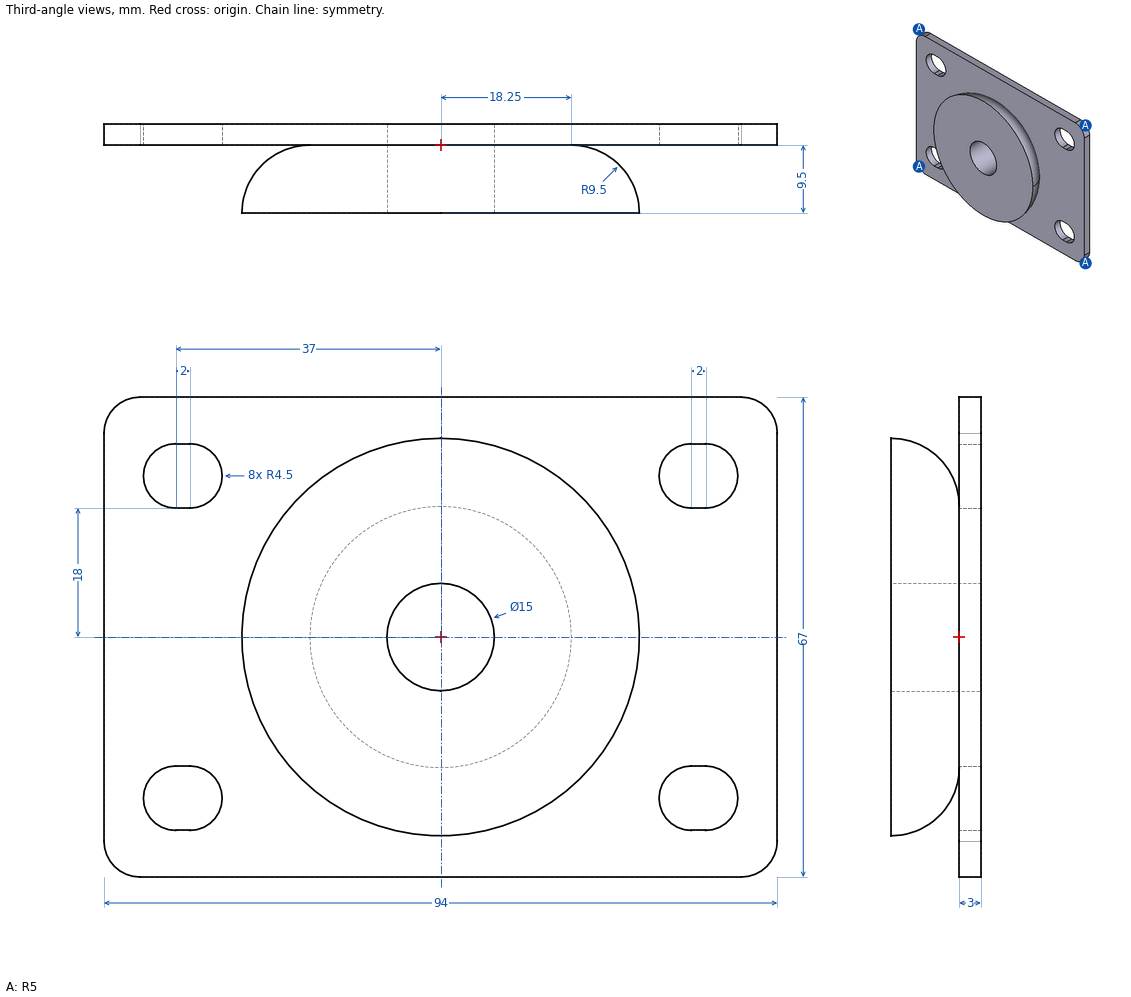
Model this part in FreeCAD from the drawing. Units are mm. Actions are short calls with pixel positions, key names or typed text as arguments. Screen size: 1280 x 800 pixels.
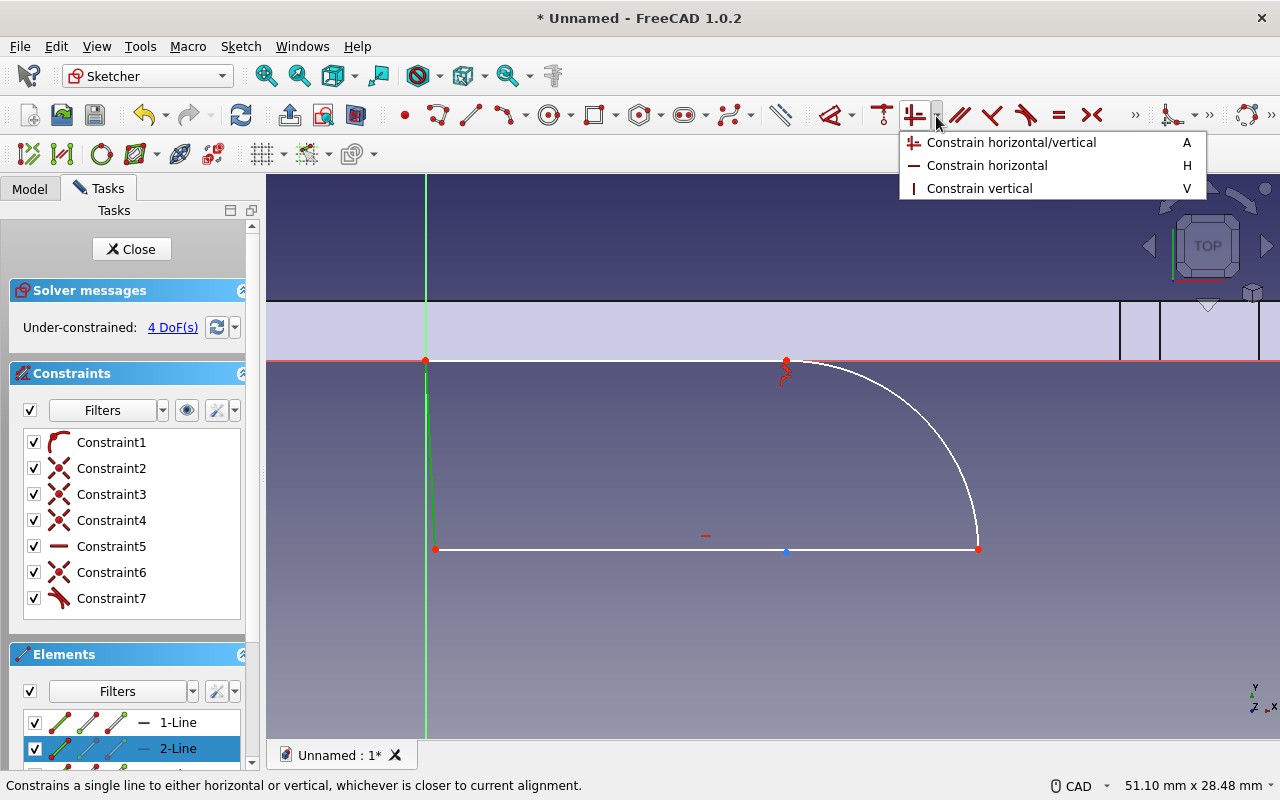
click(1053, 188)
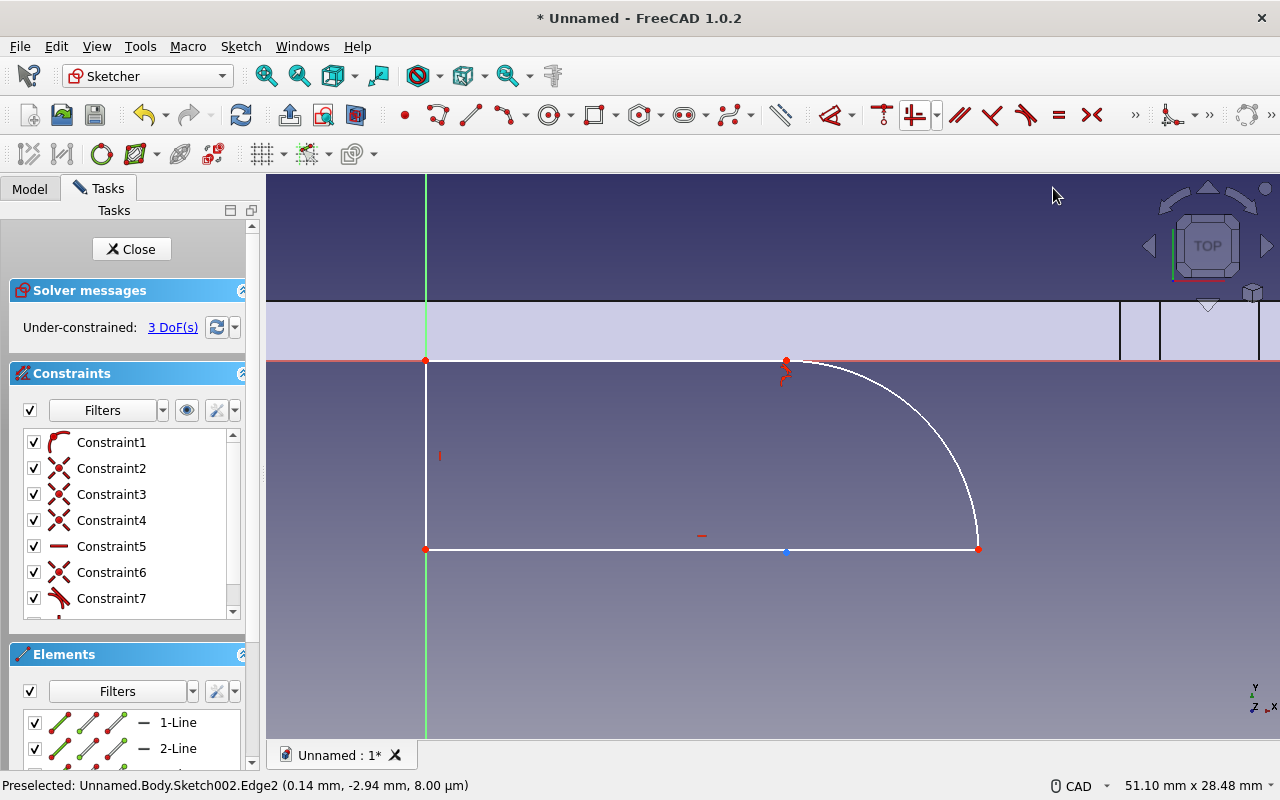
key(d)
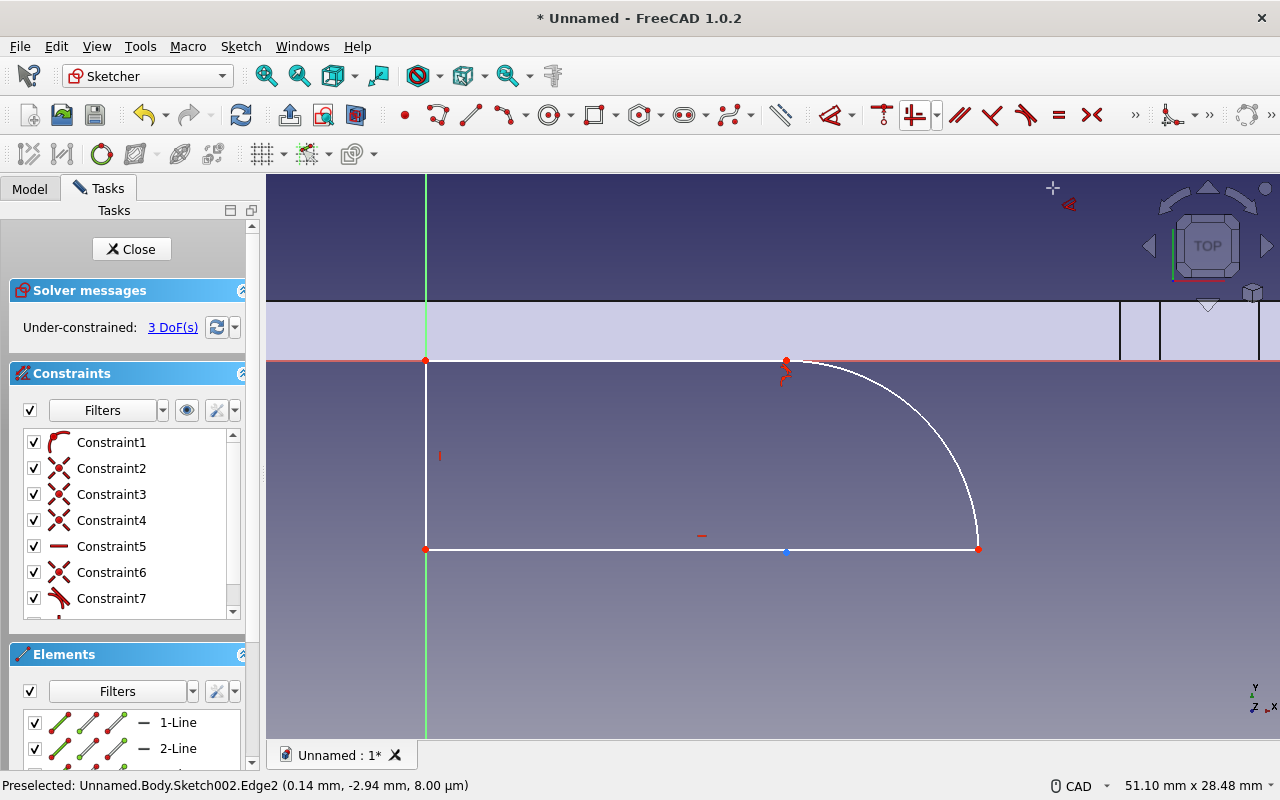
click(957, 464)
click(985, 449)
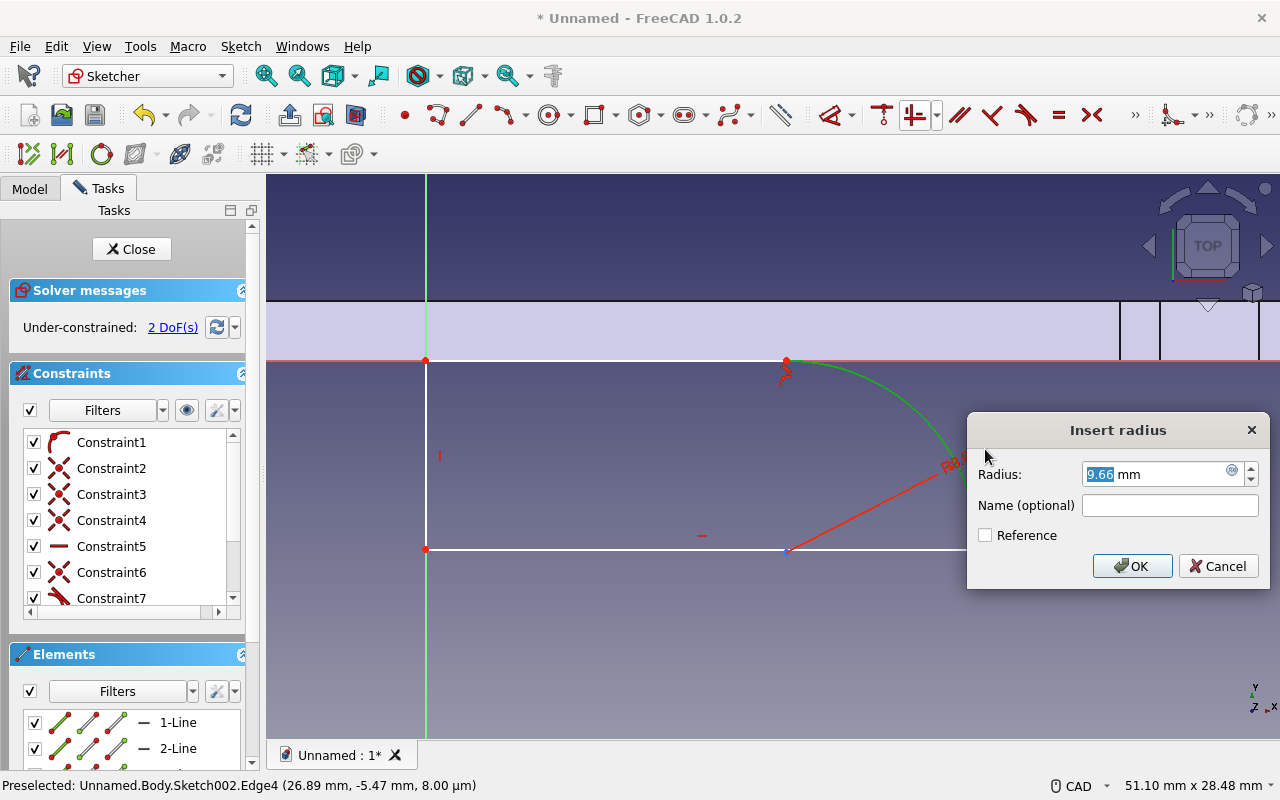
text(9.5)
key(Return)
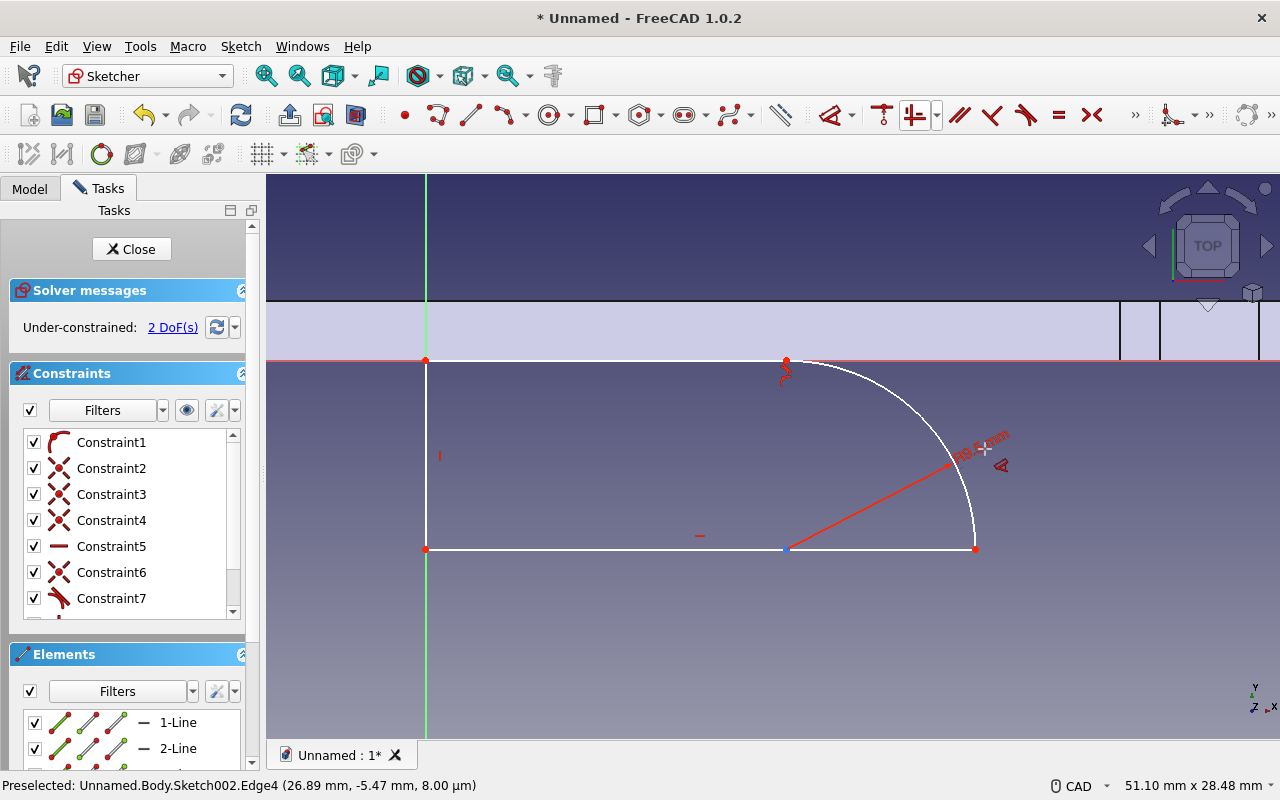
click(426, 418)
click(392, 455)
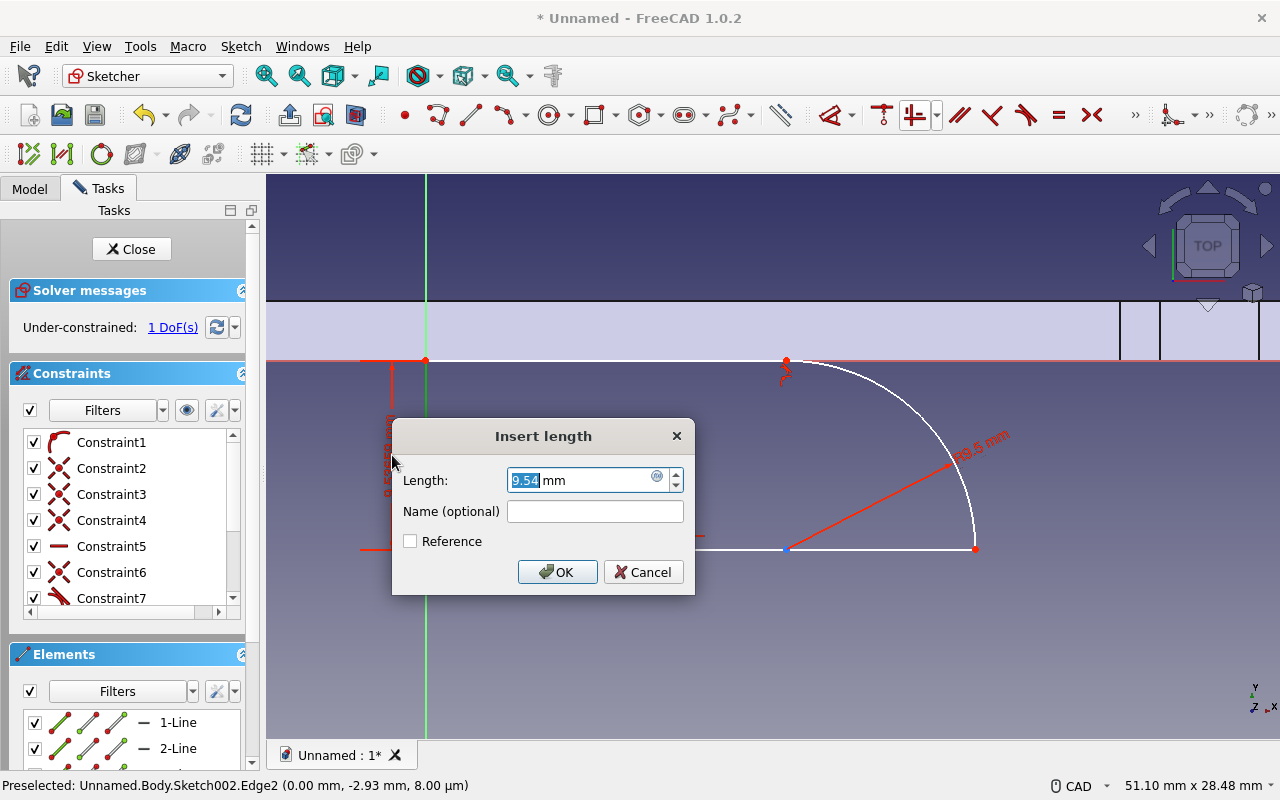
text(9.5)
key(Return)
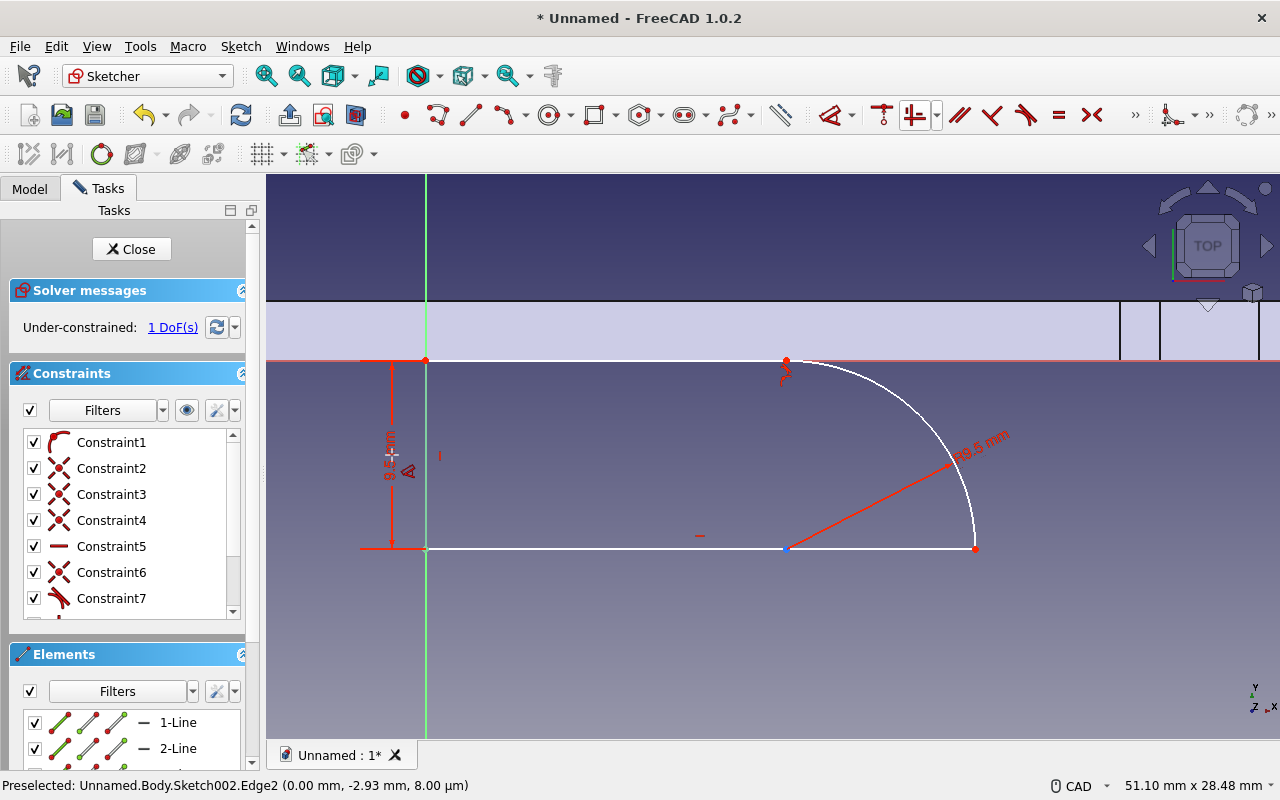
click(679, 361)
click(606, 327)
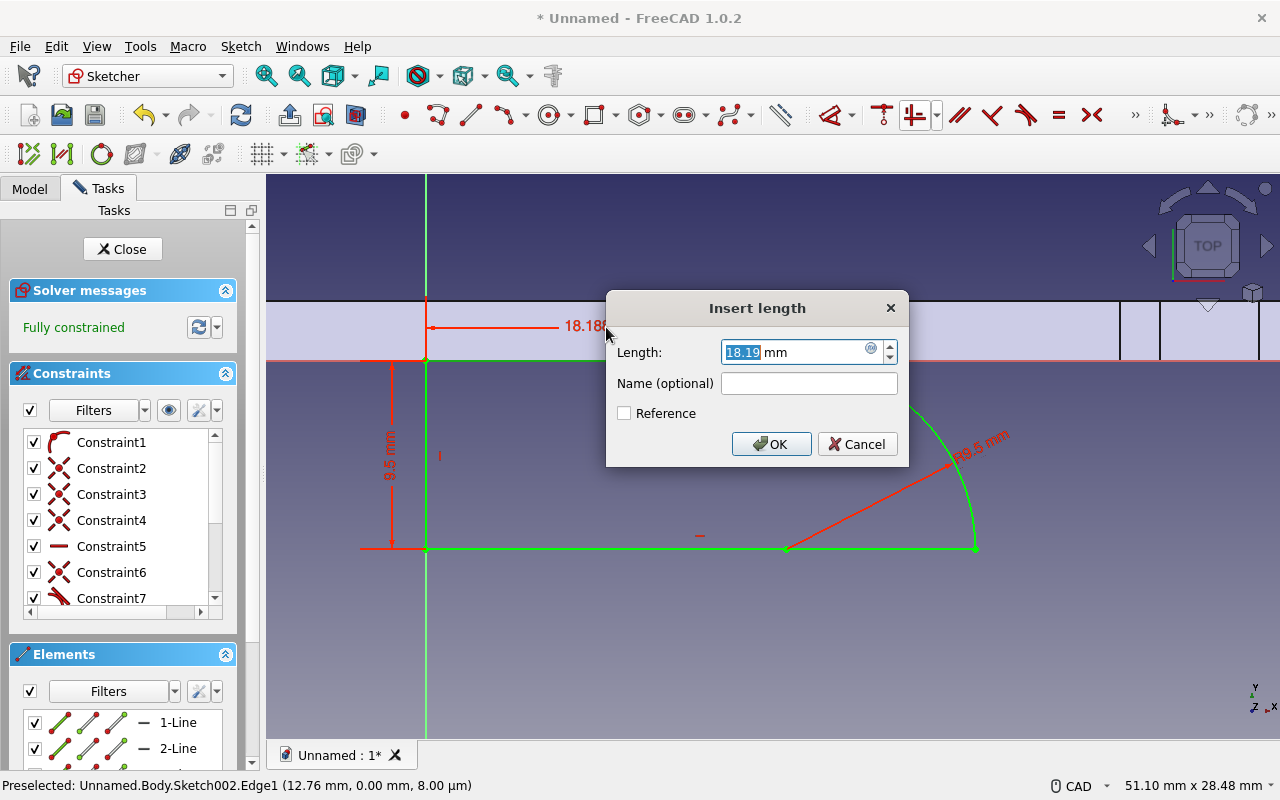
text(18.25)
key(Return)
key(Escape)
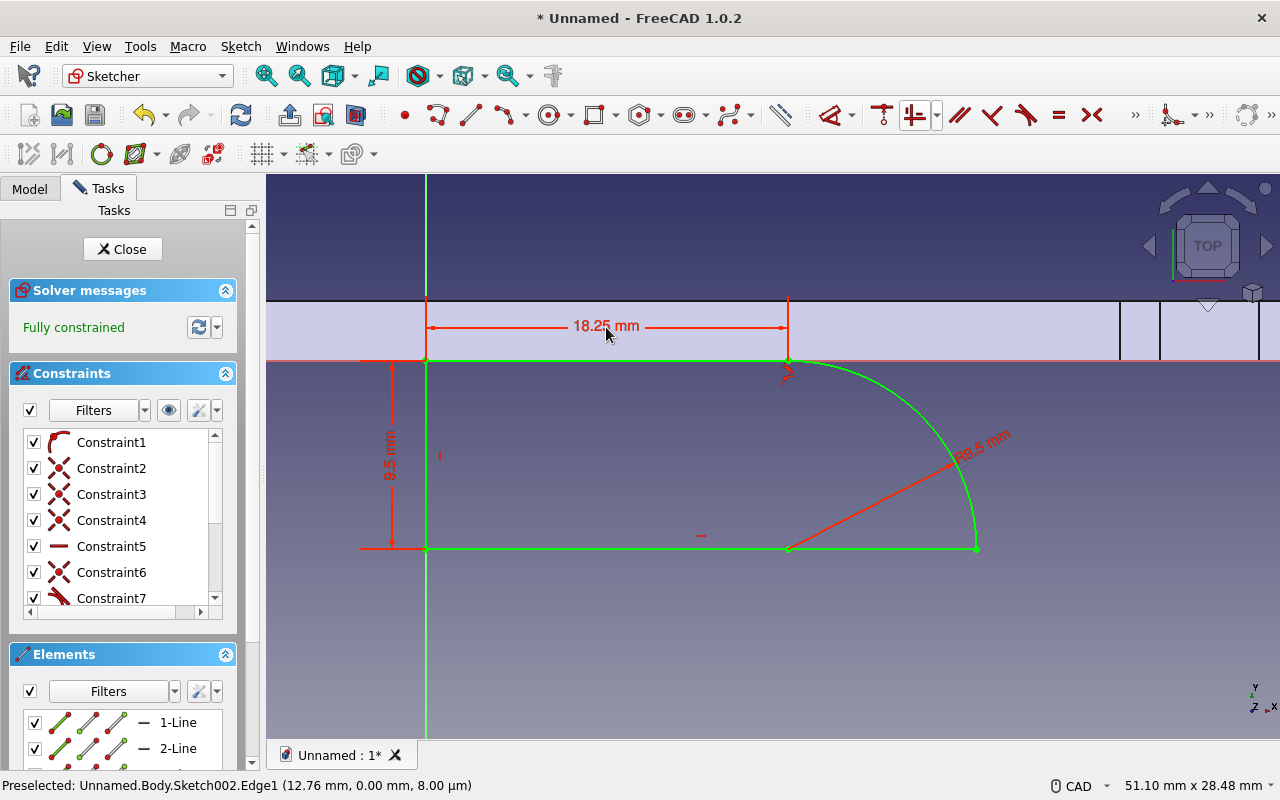
click(123, 249)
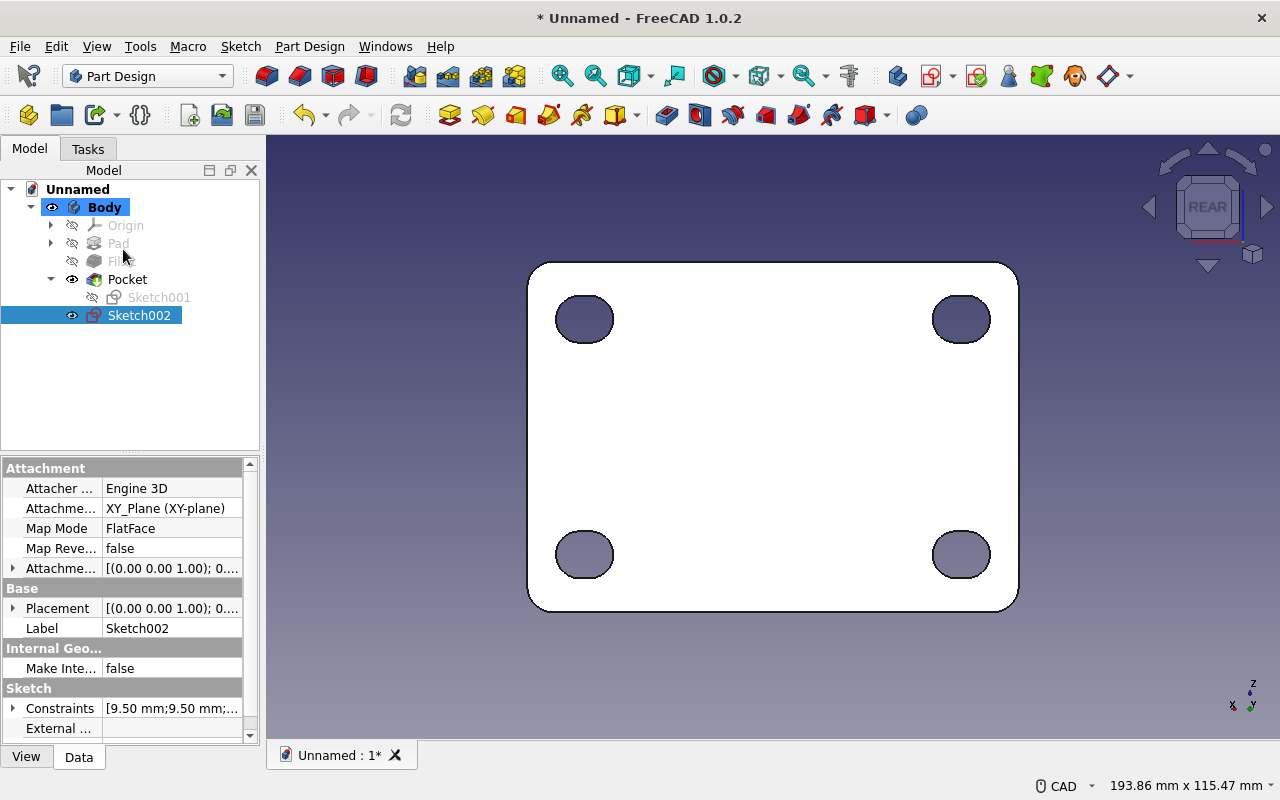
click(483, 116)